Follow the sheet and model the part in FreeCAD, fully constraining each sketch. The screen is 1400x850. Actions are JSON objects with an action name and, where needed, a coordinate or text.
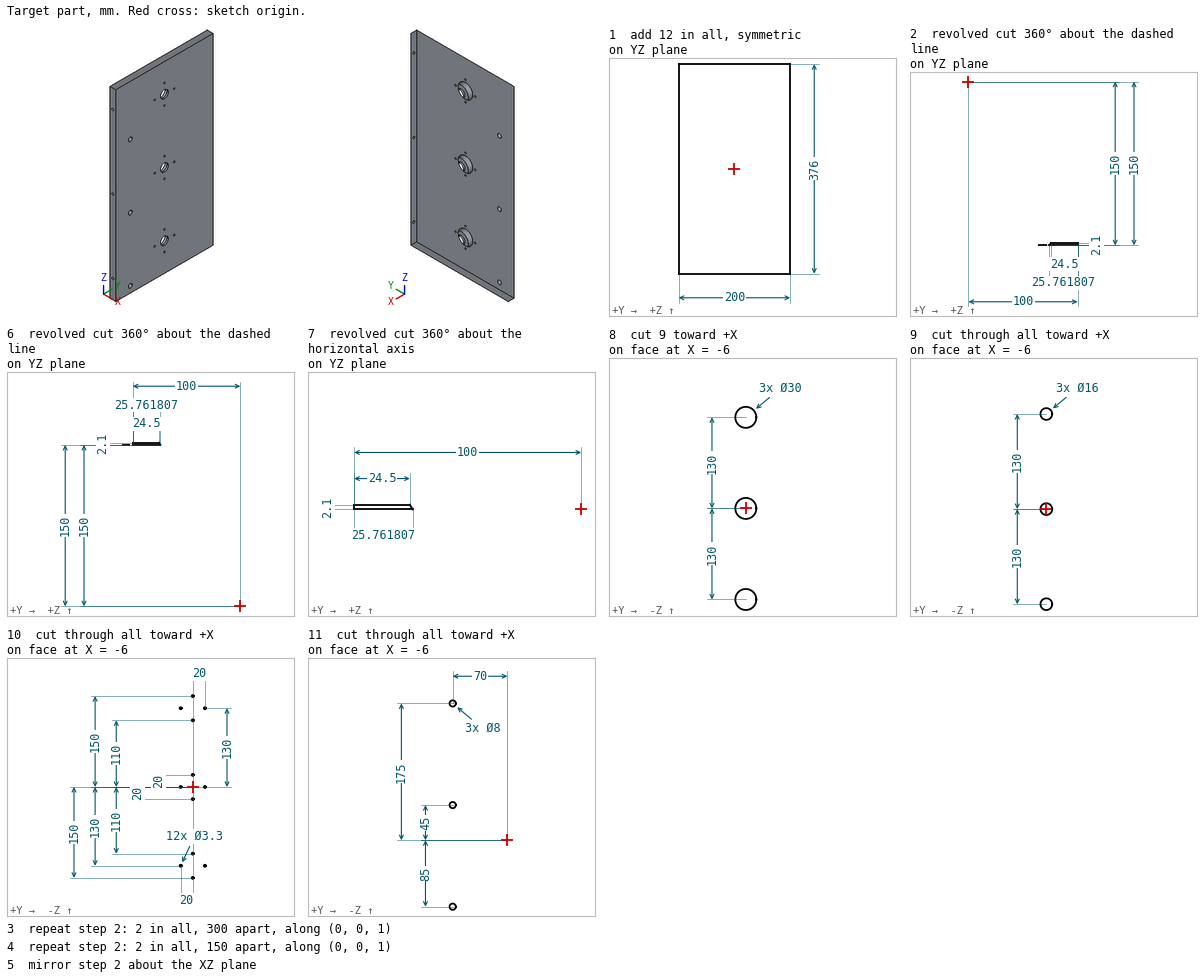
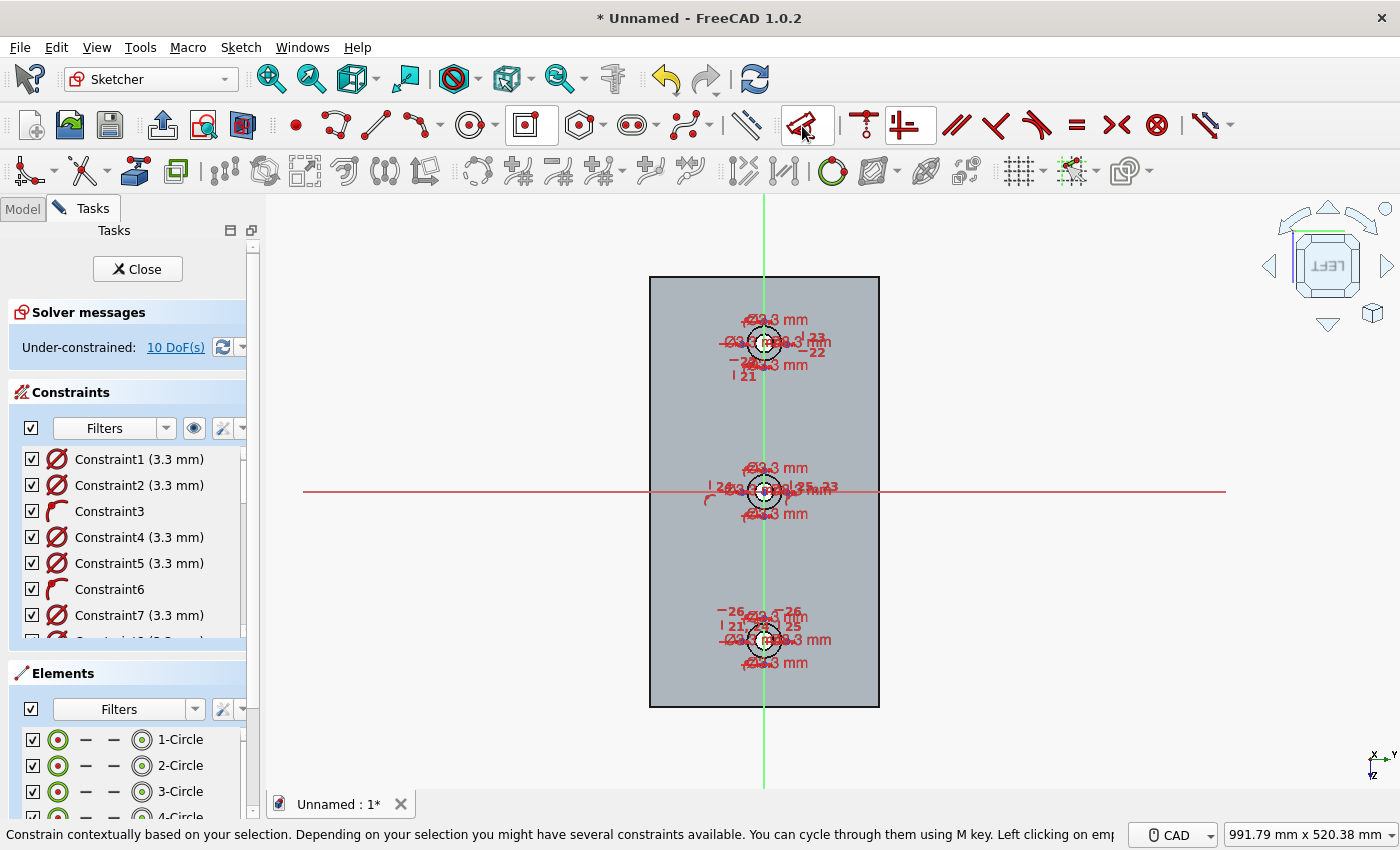
{"action": "scroll", "coordinate": [742, 642], "scroll_direction": "up", "scroll_amount": 3}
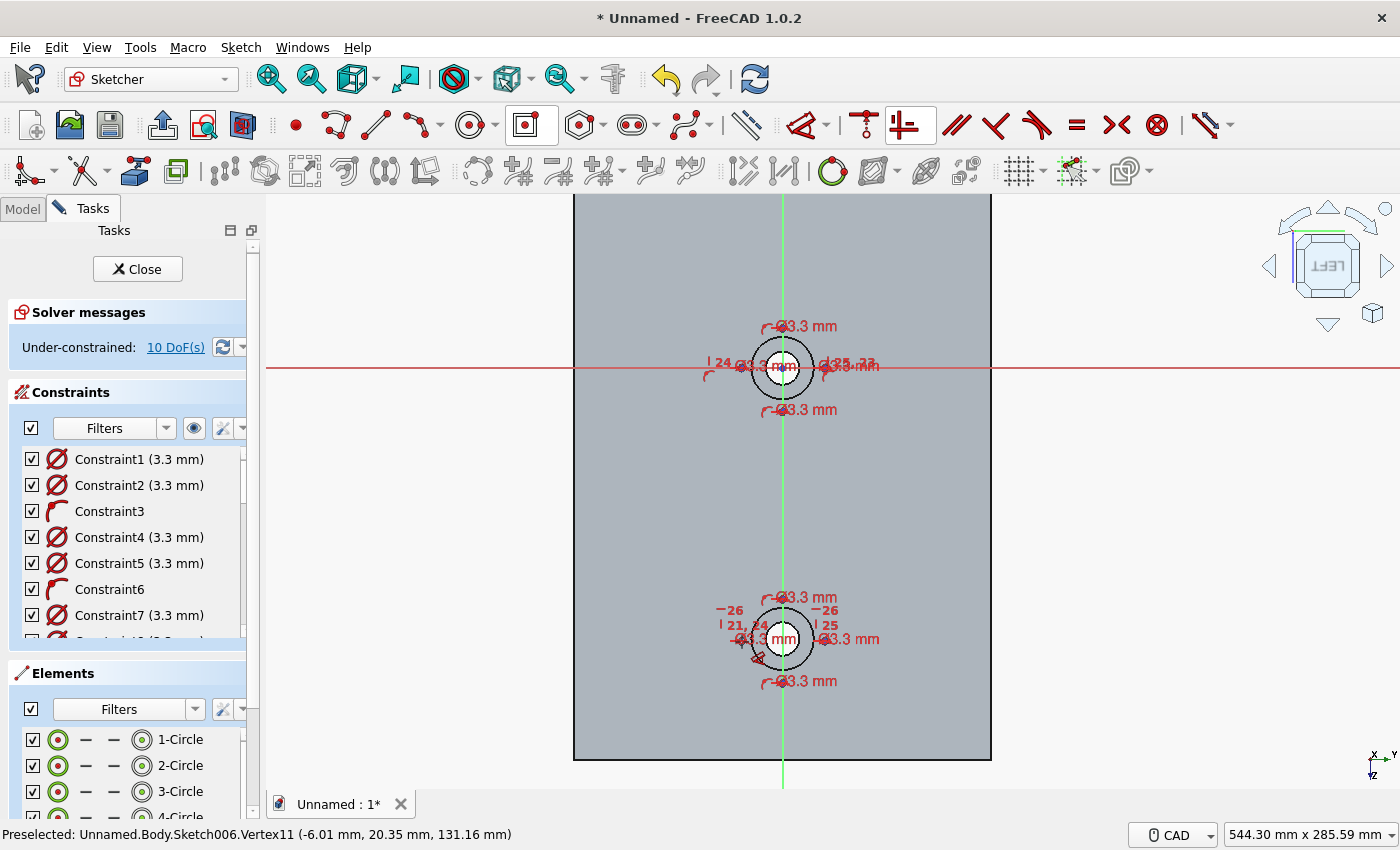
{"action": "left_click", "coordinate": [742, 641]}
{"action": "left_click", "coordinate": [762, 675]}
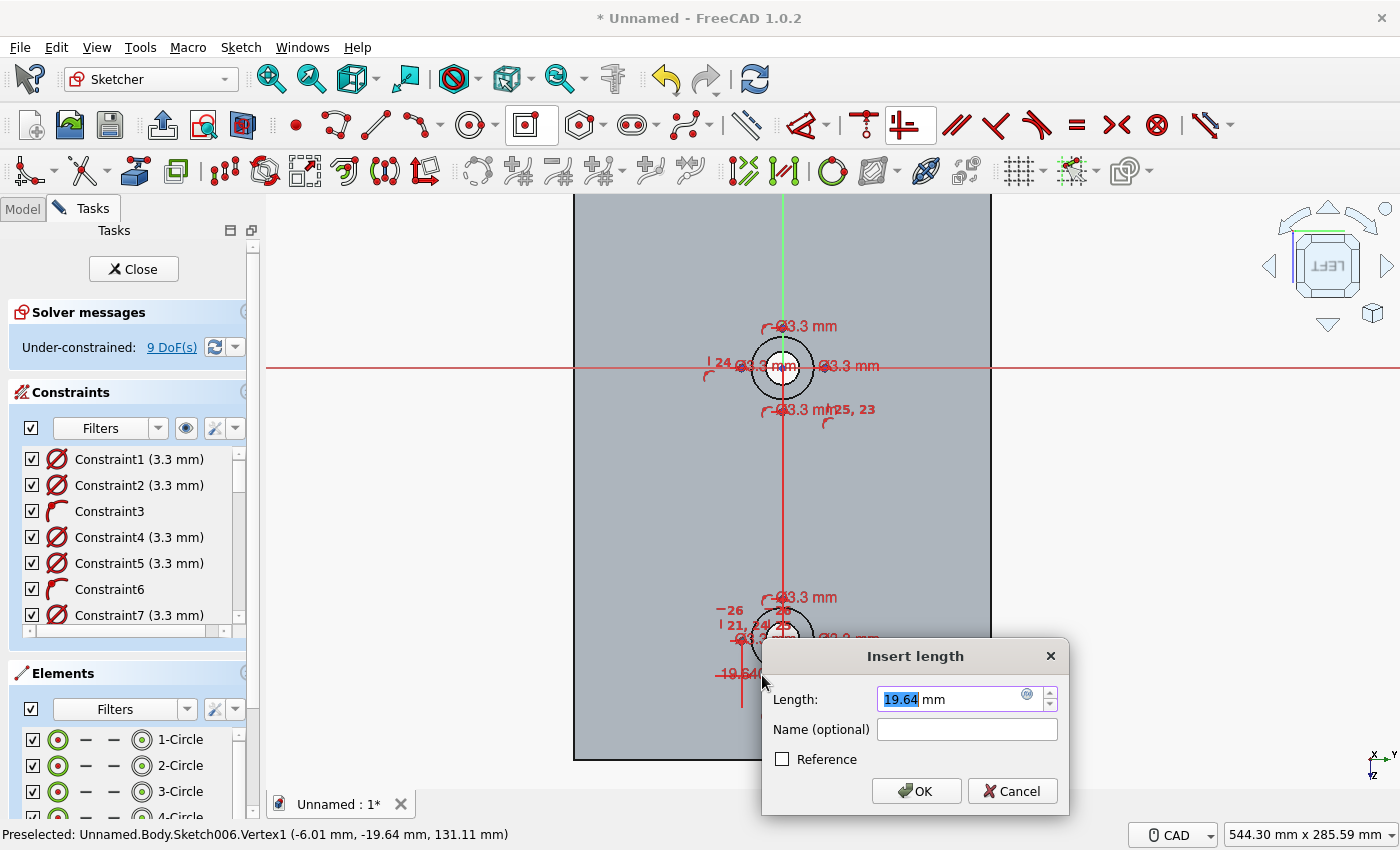
{"action": "type", "text": "20"}
{"action": "key", "text": "Return"}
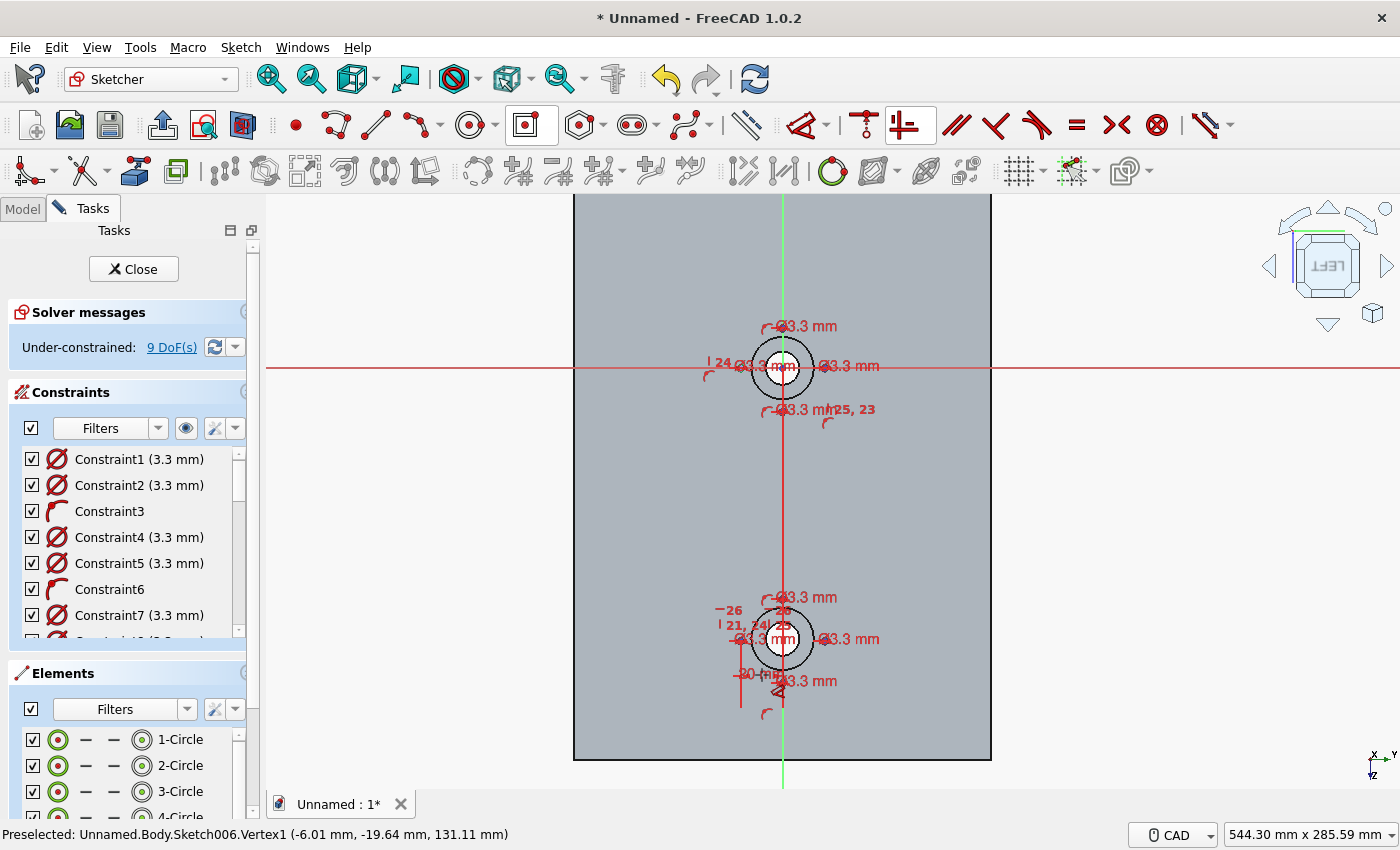
{"action": "scroll", "coordinate": [743, 642], "scroll_direction": "down", "scroll_amount": 3}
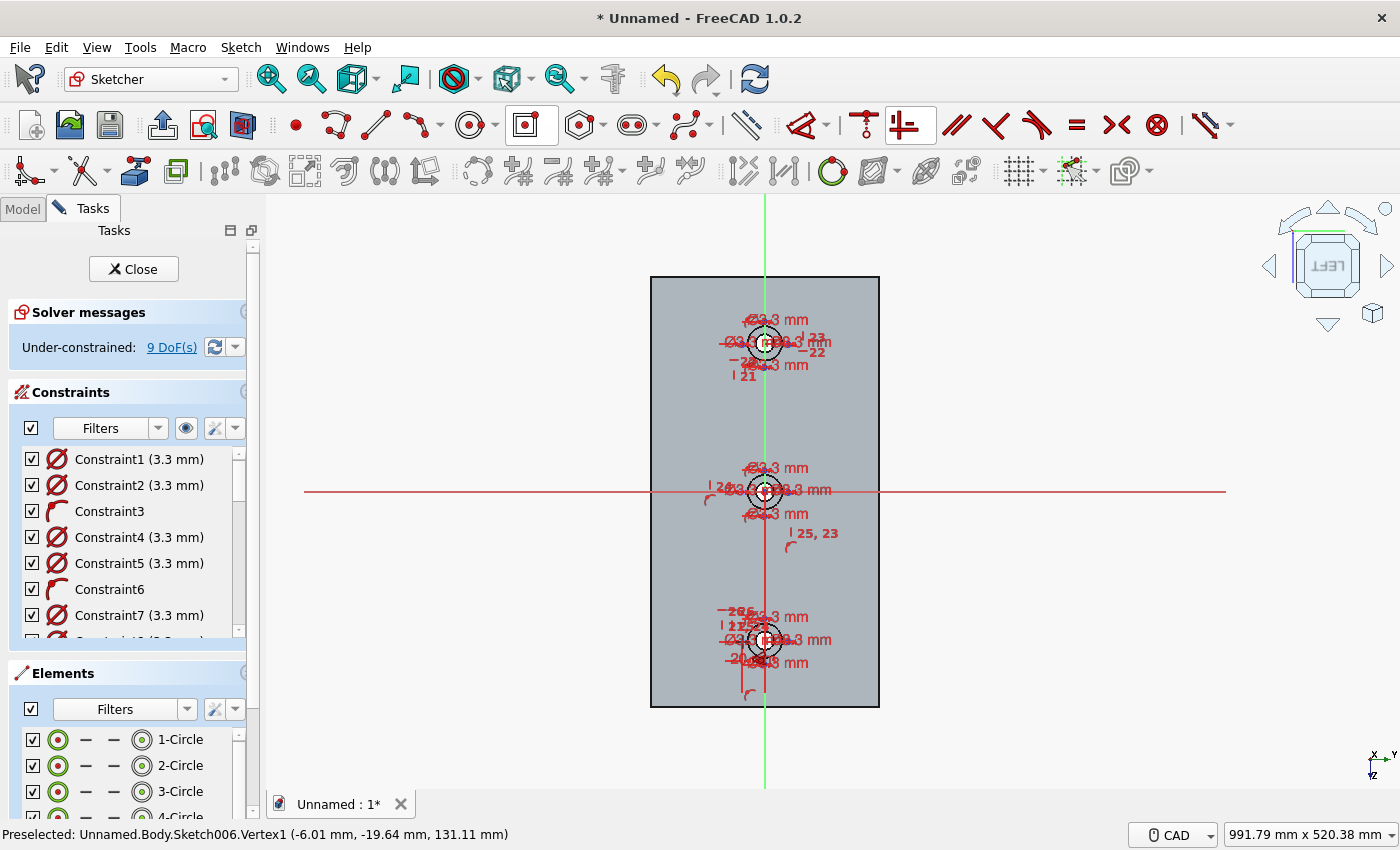
{"action": "scroll", "coordinate": [788, 344], "scroll_direction": "up", "scroll_amount": 3}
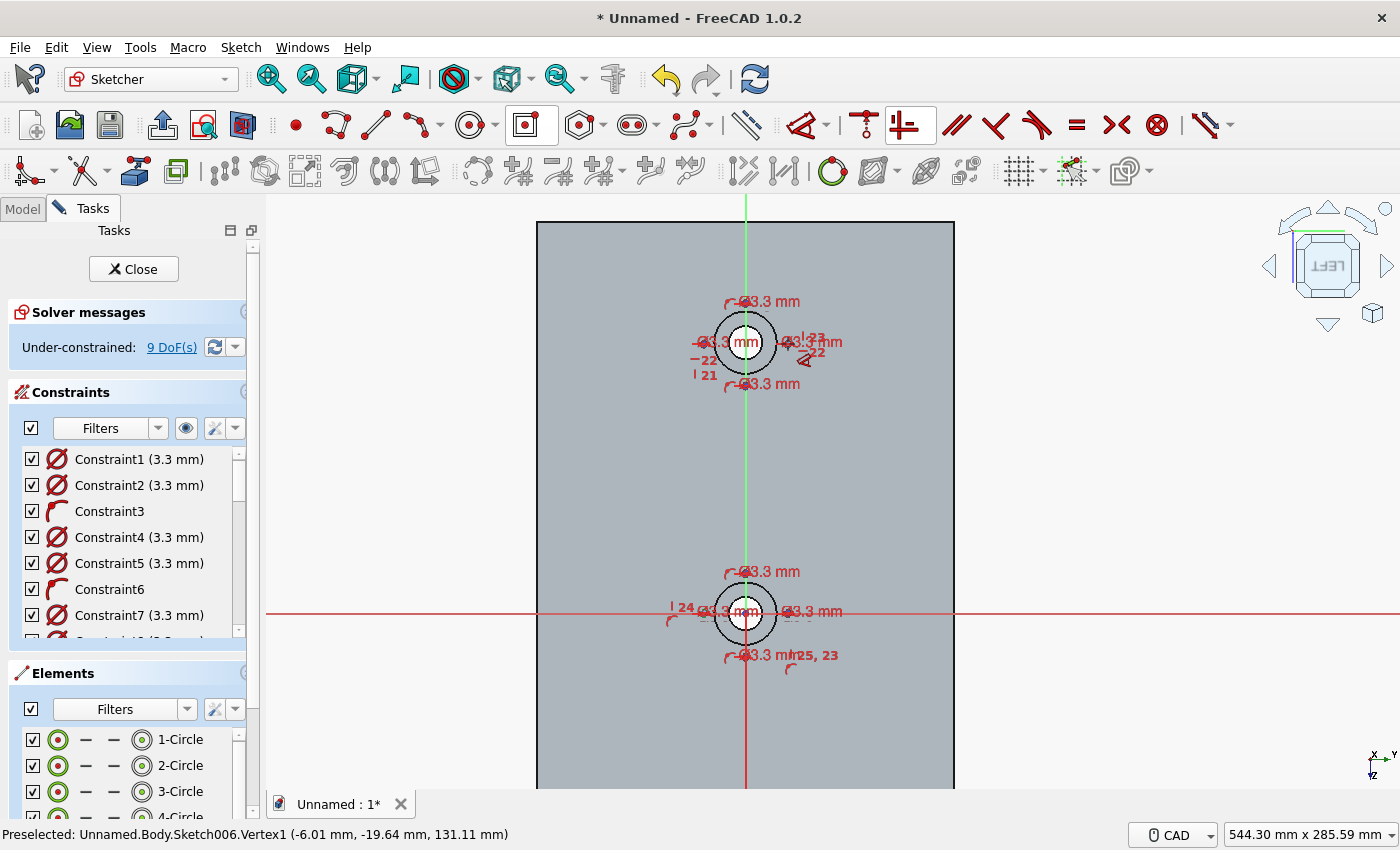
{"action": "left_click", "coordinate": [788, 344]}
{"action": "left_click", "coordinate": [767, 310]}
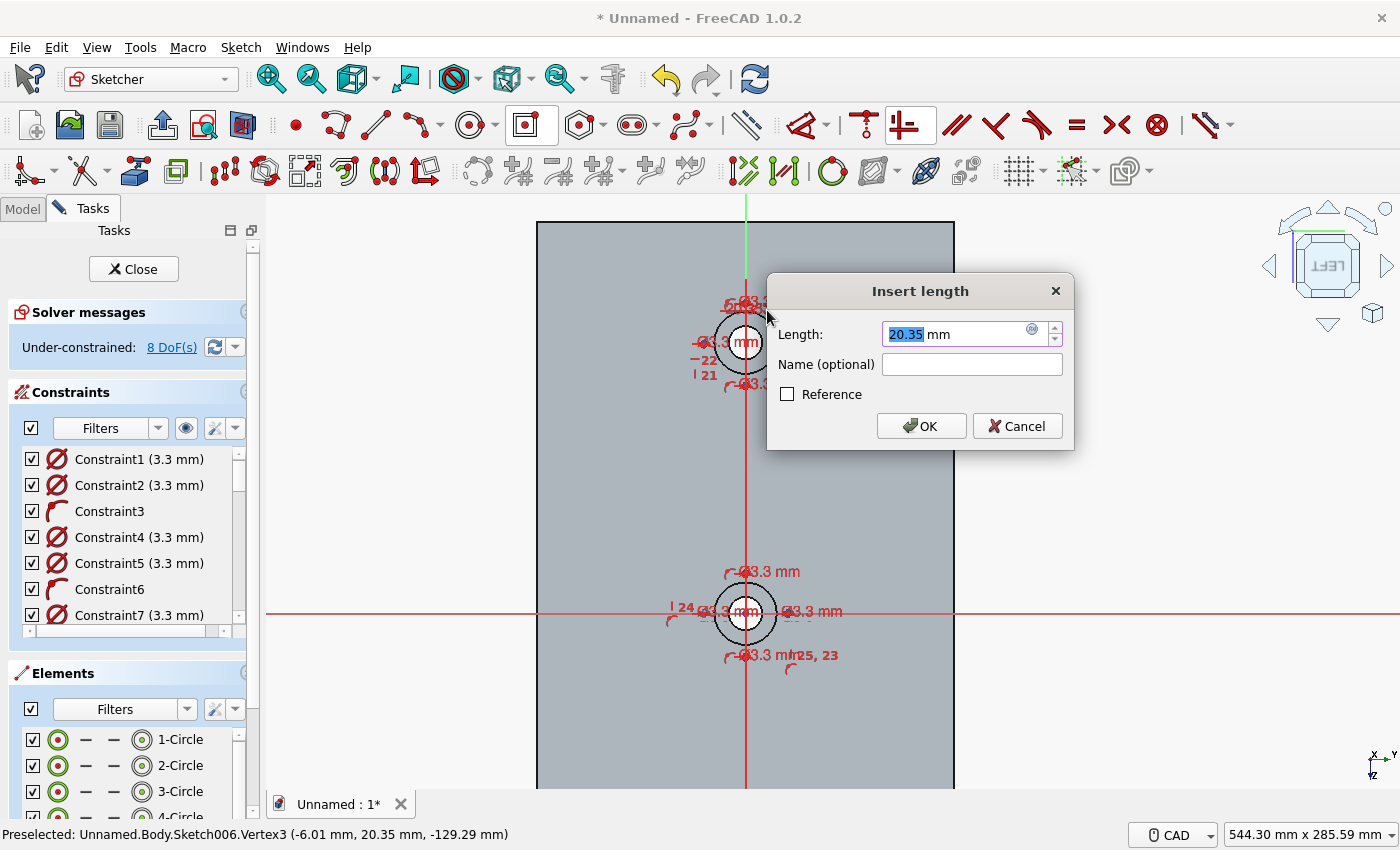
{"action": "type", "text": "20"}
{"action": "key", "text": "Return"}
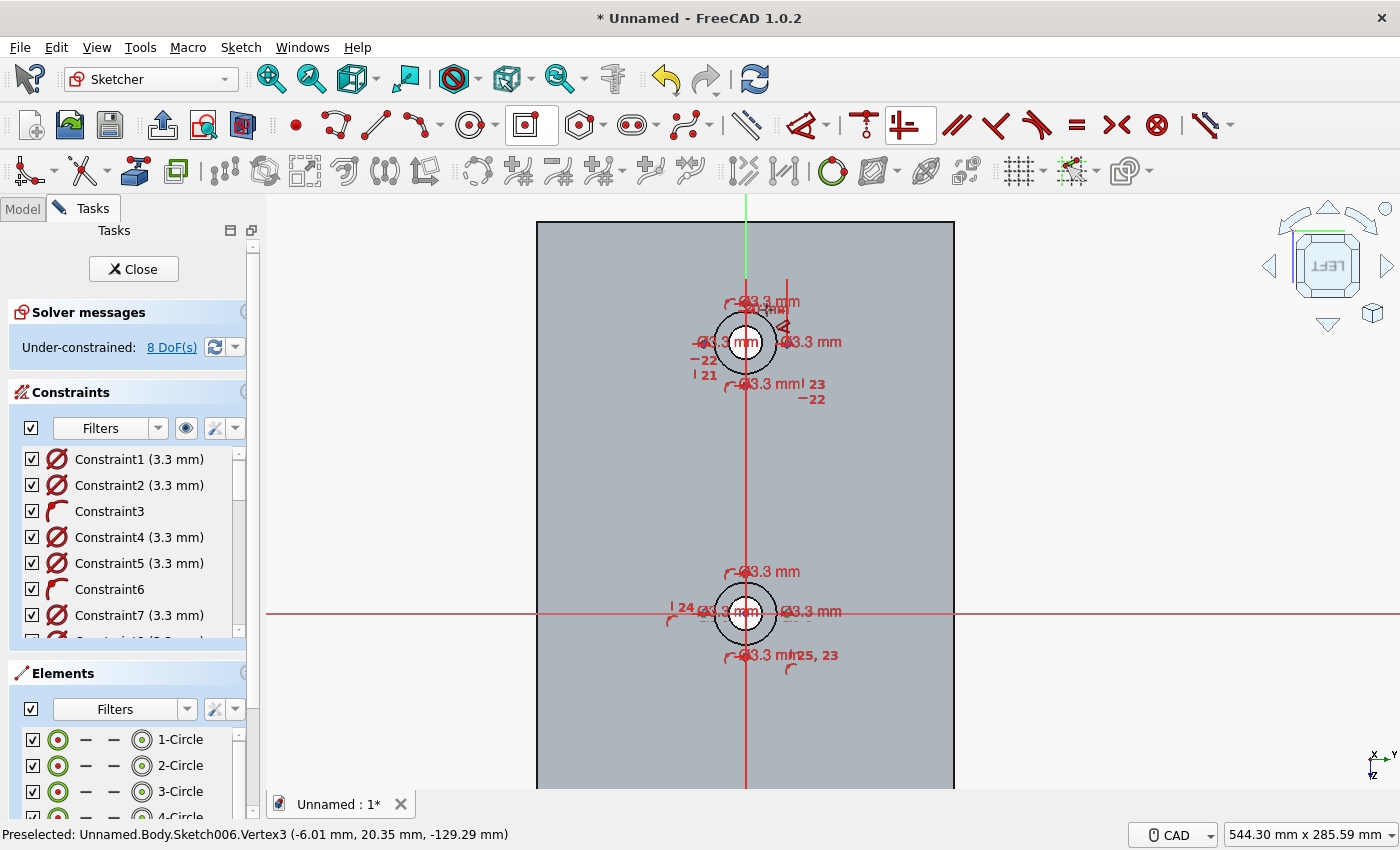
{"action": "left_click", "coordinate": [746, 574]}
{"action": "left_click", "coordinate": [780, 594]}